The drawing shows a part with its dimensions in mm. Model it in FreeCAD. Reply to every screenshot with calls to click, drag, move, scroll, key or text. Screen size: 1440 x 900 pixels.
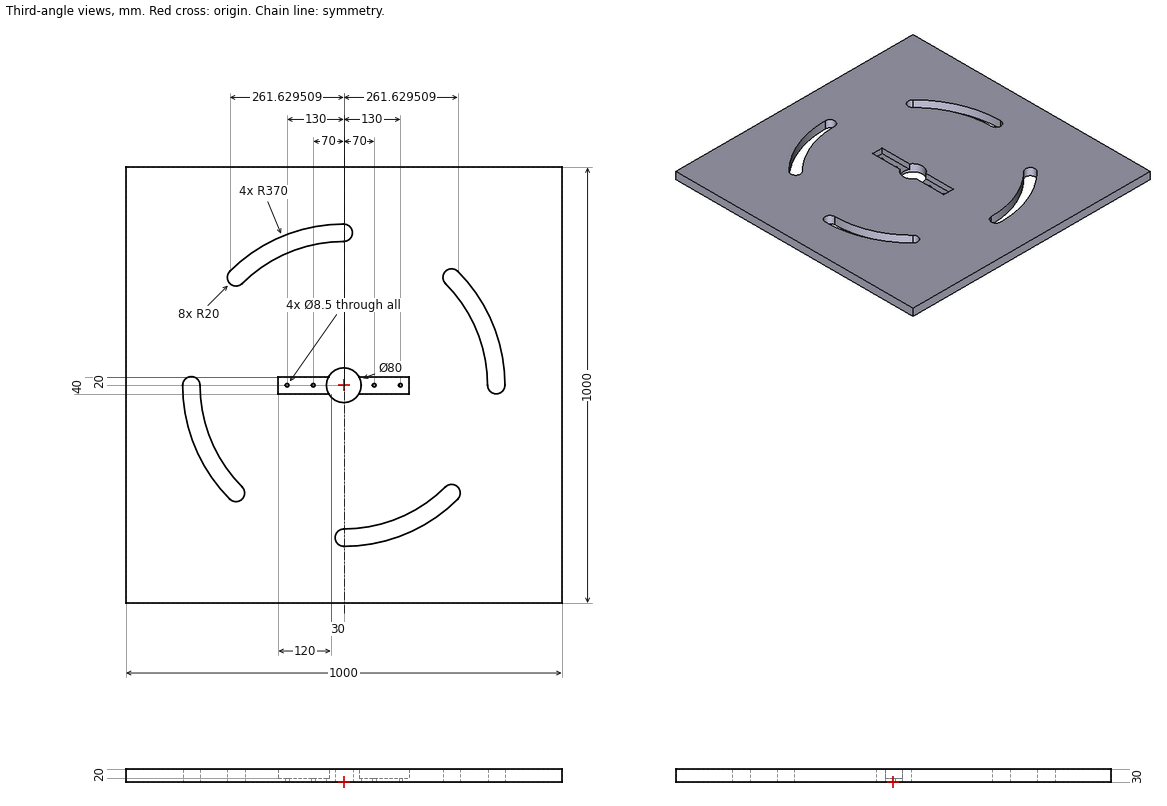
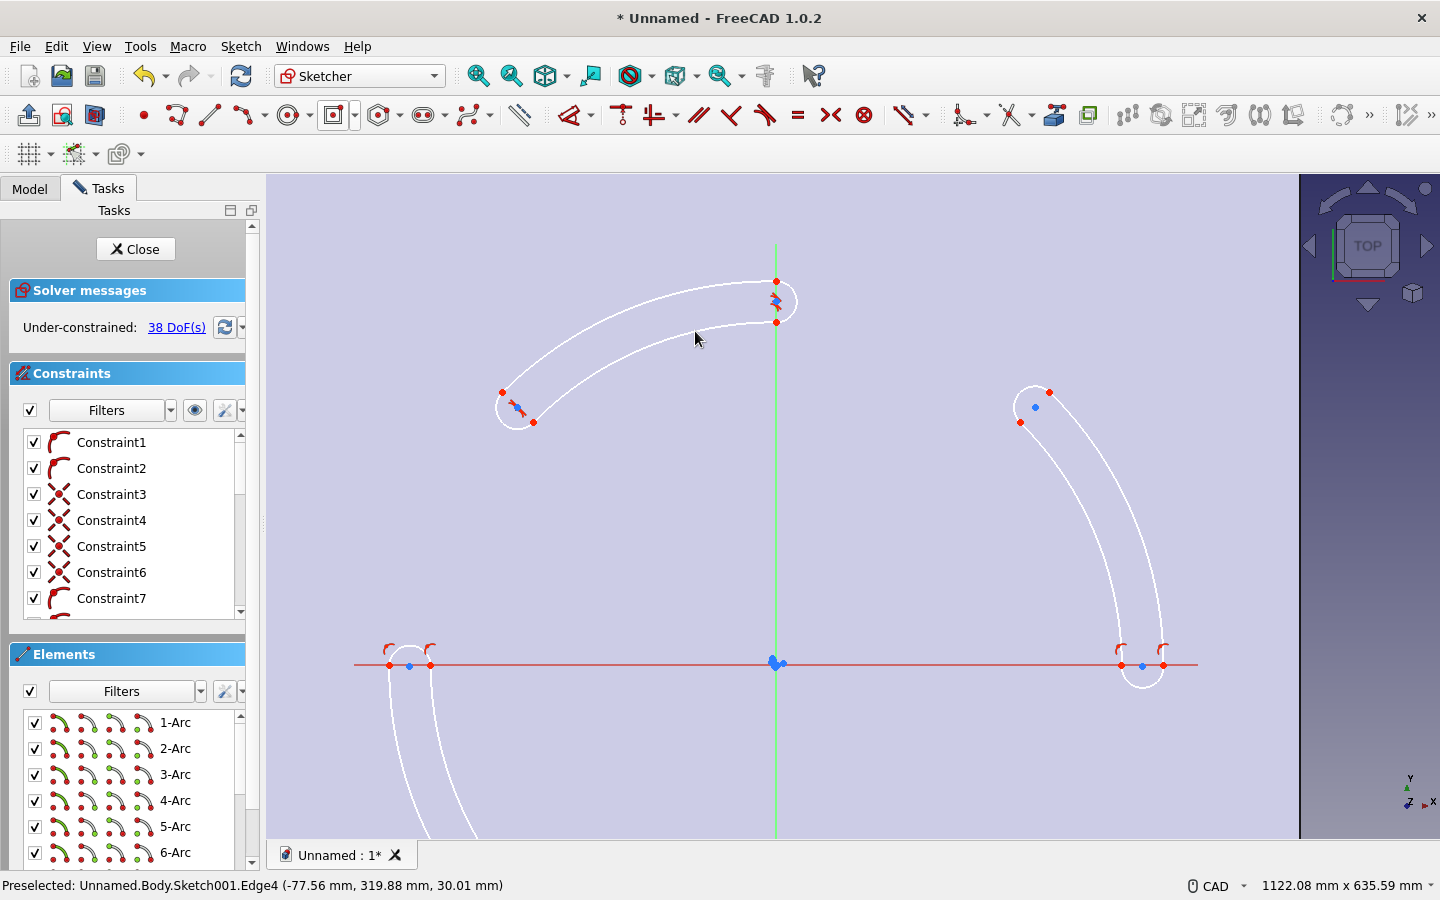
click(1130, 683)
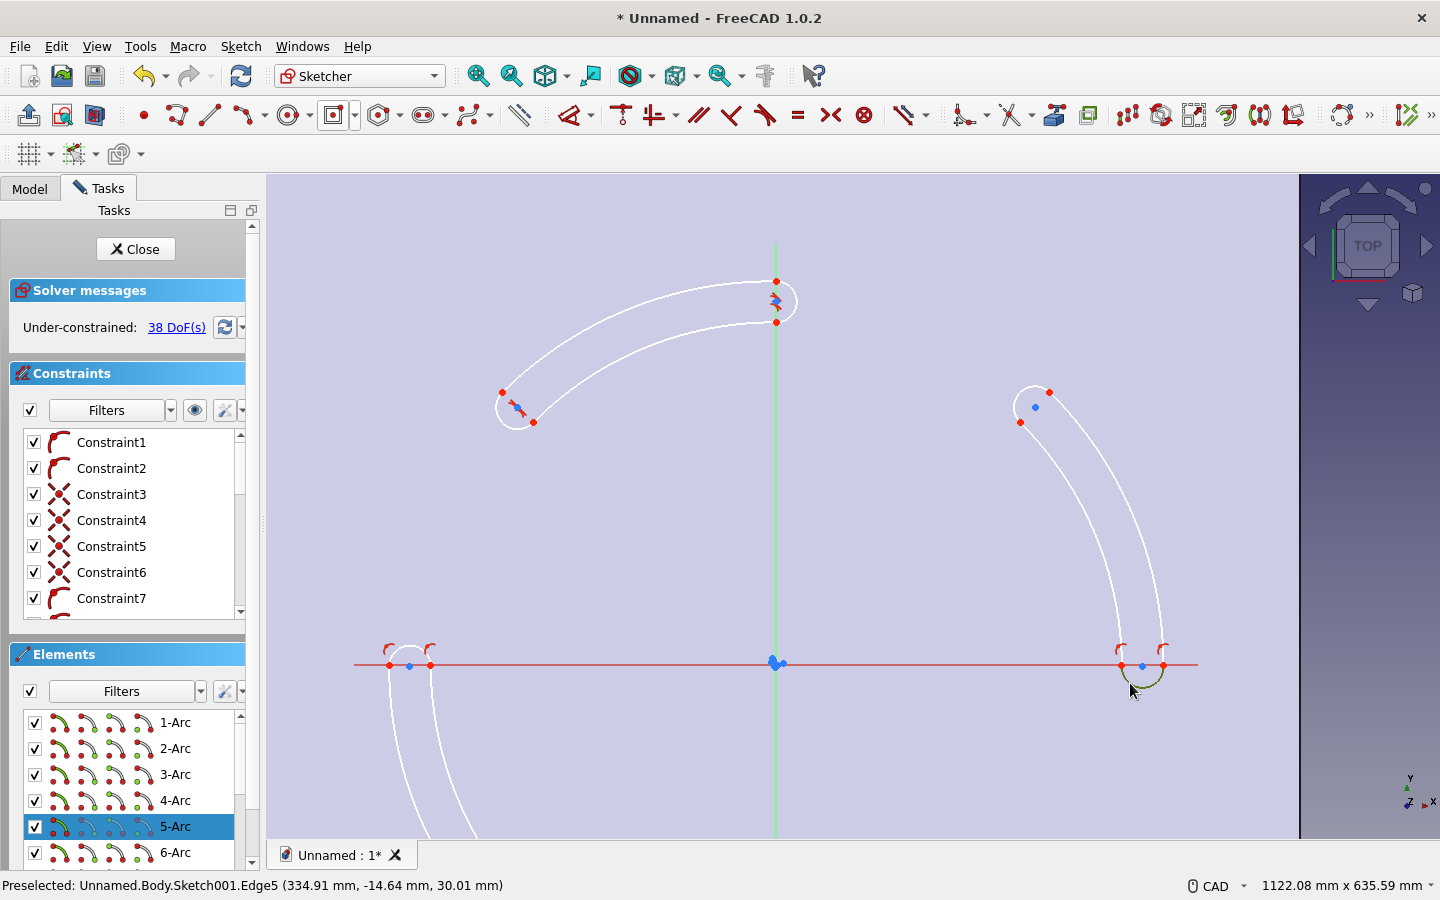
click(1153, 575)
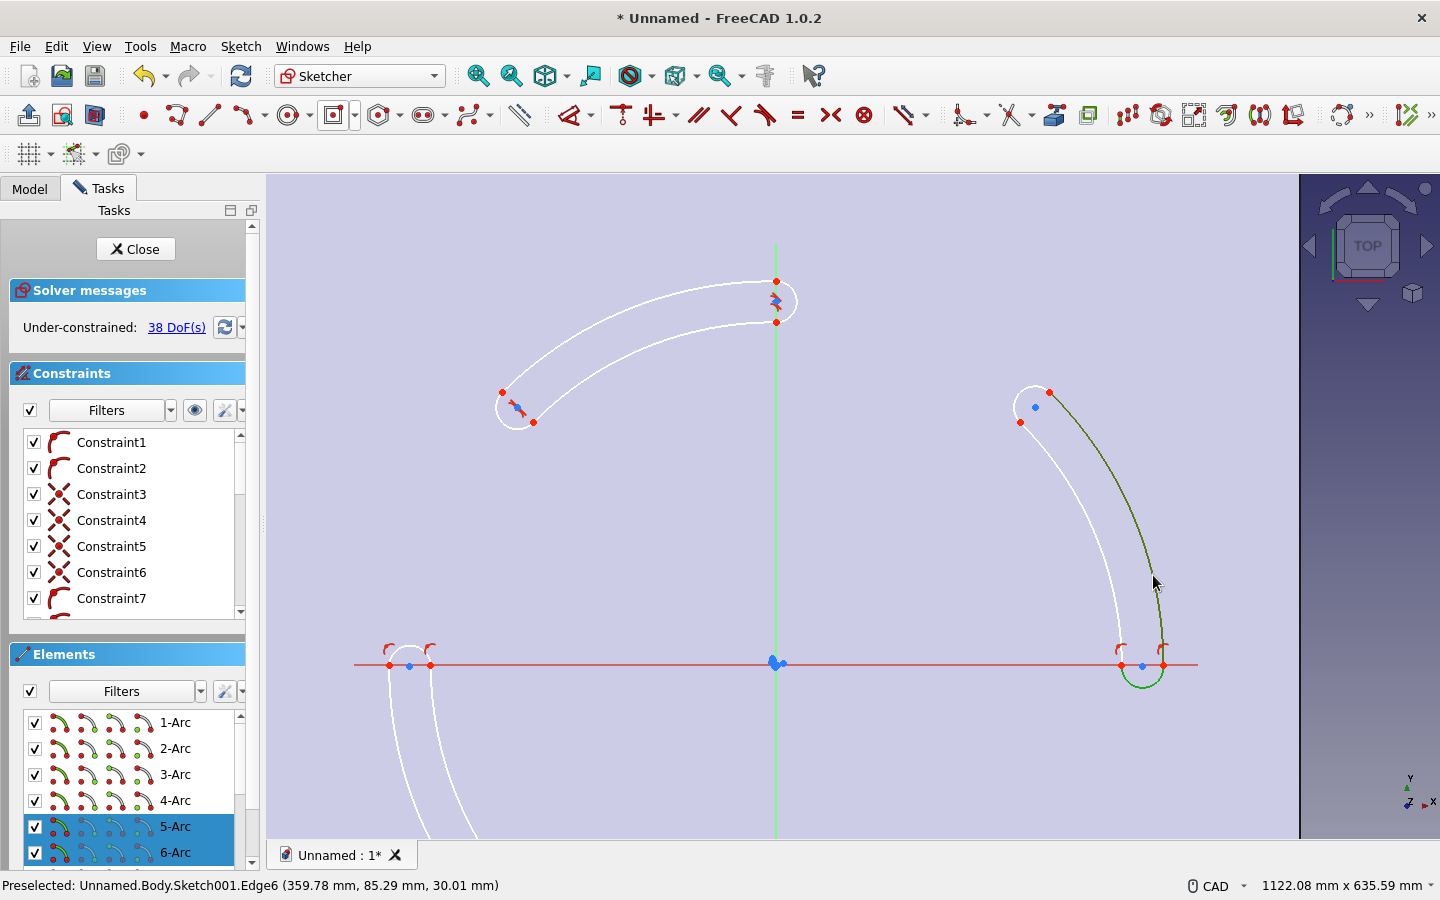
click(765, 116)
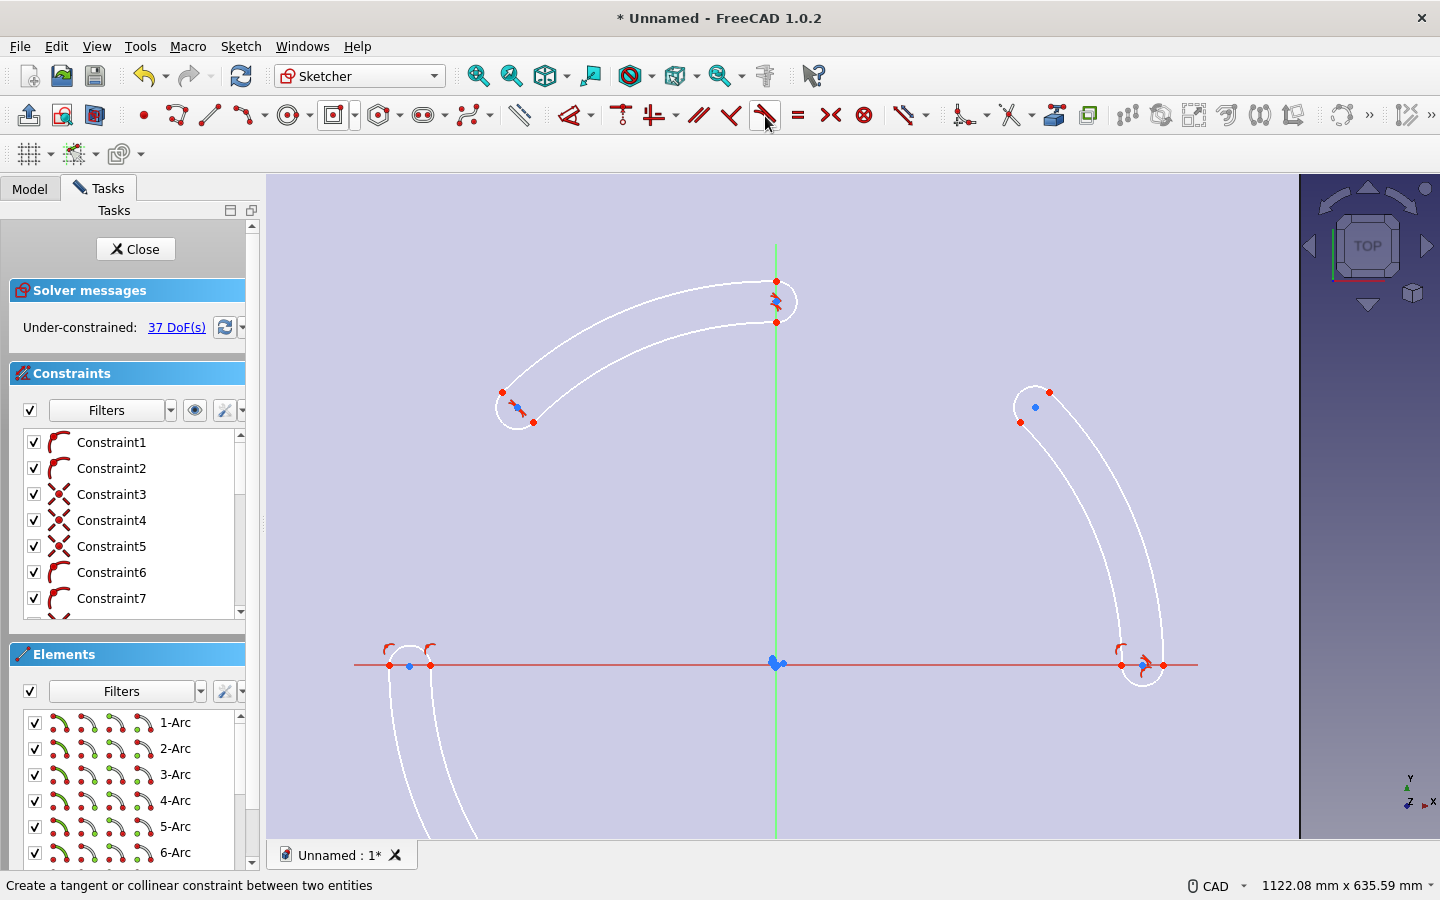
click(1153, 575)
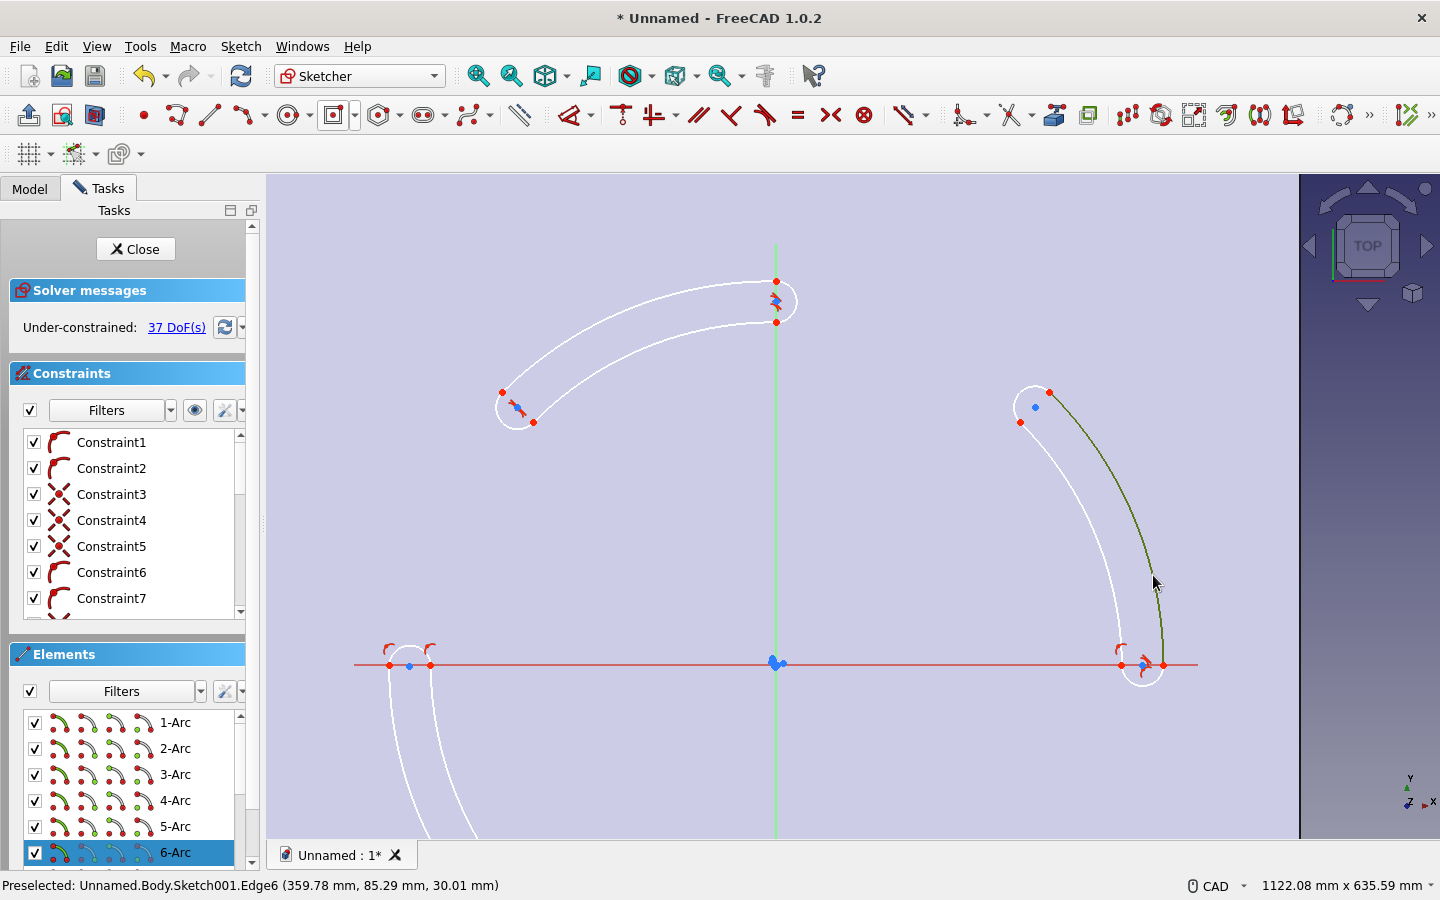
click(1031, 387)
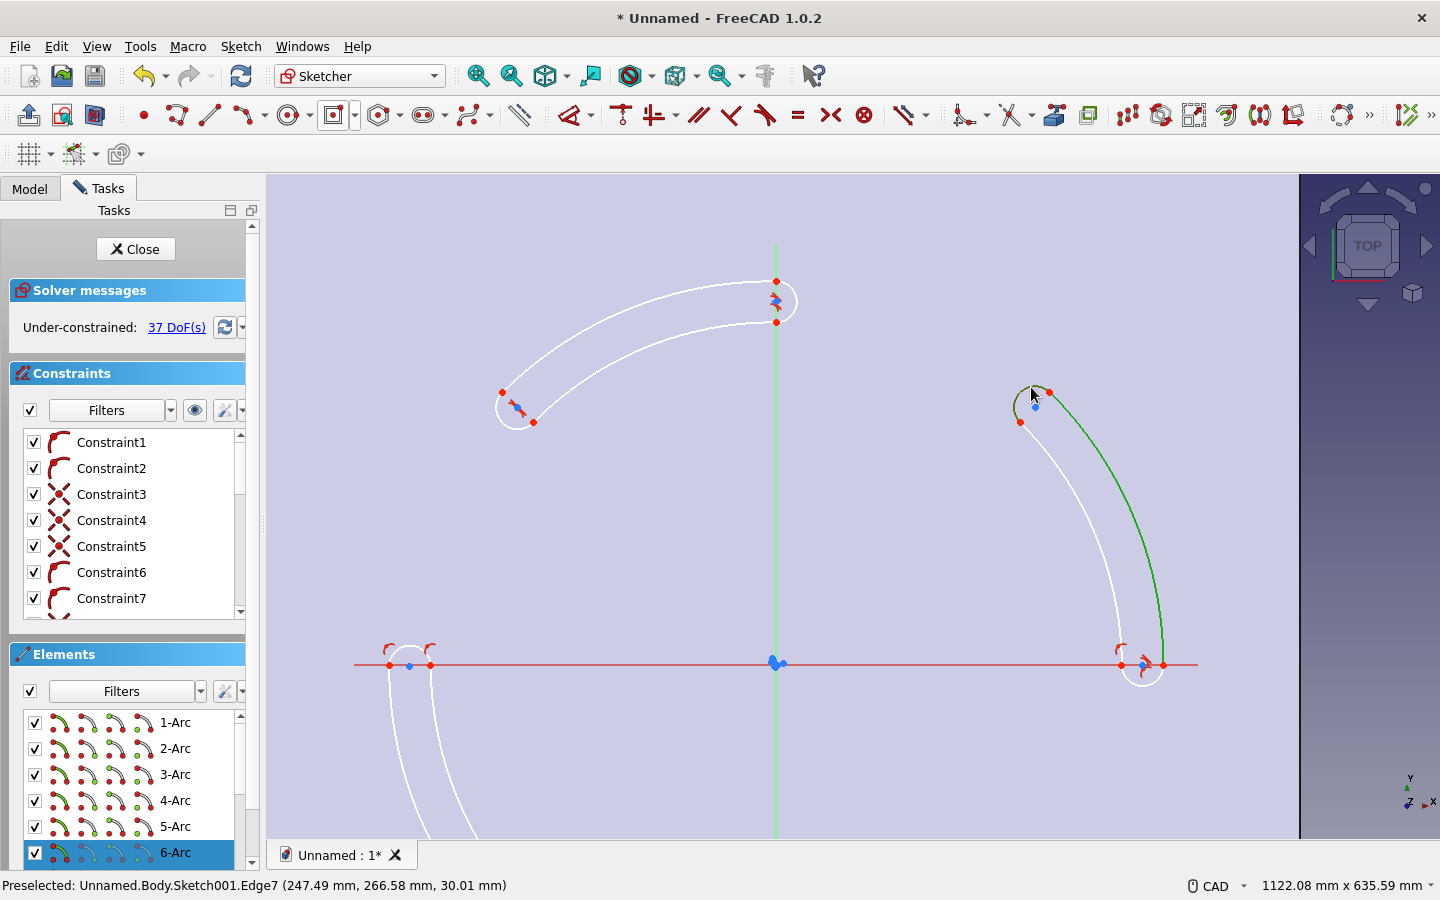
click(765, 116)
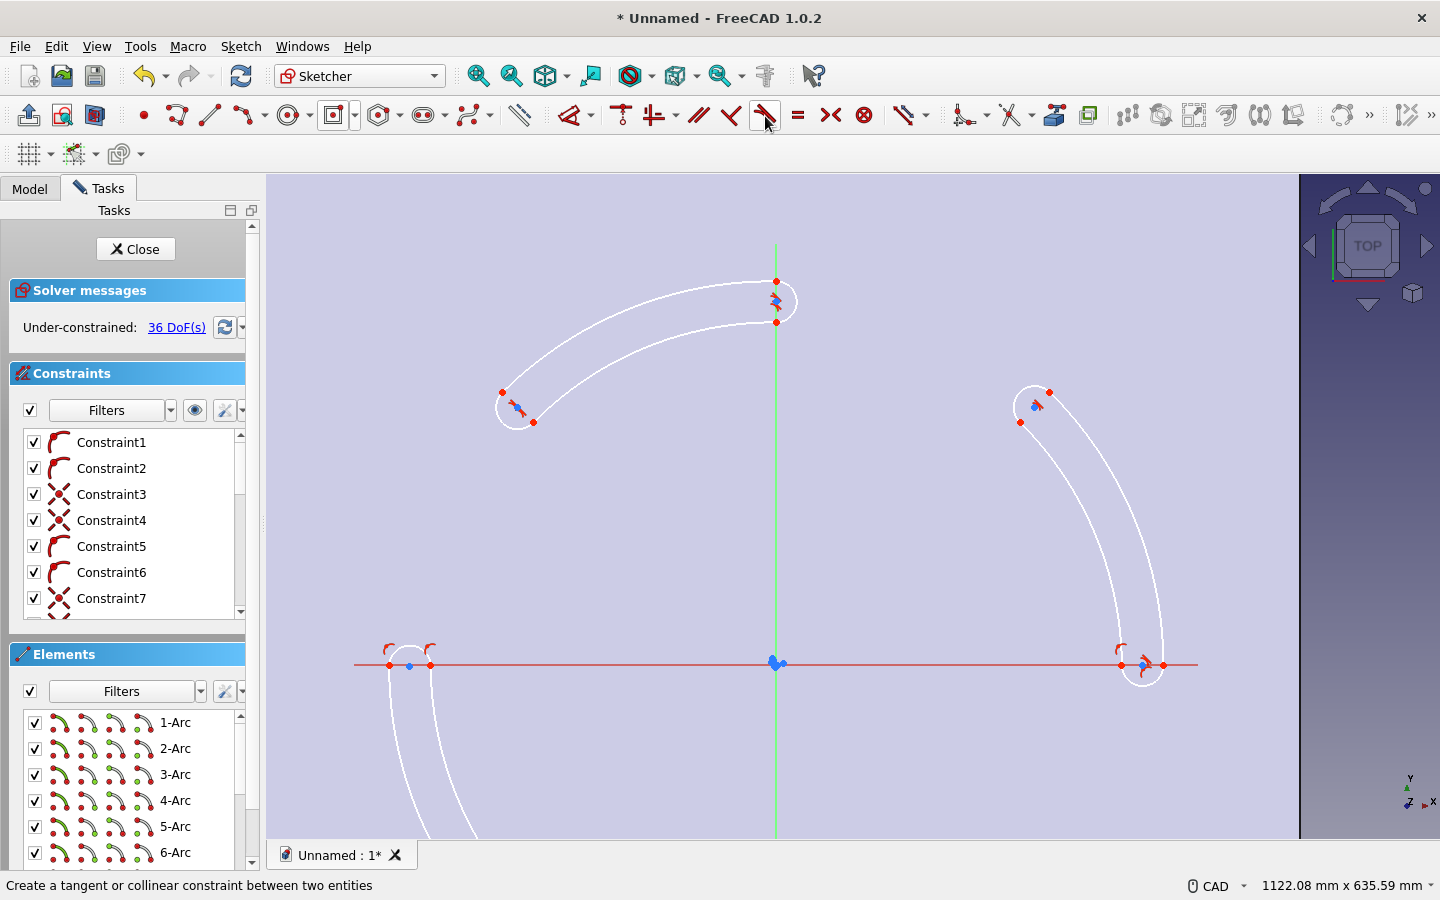
click(1031, 386)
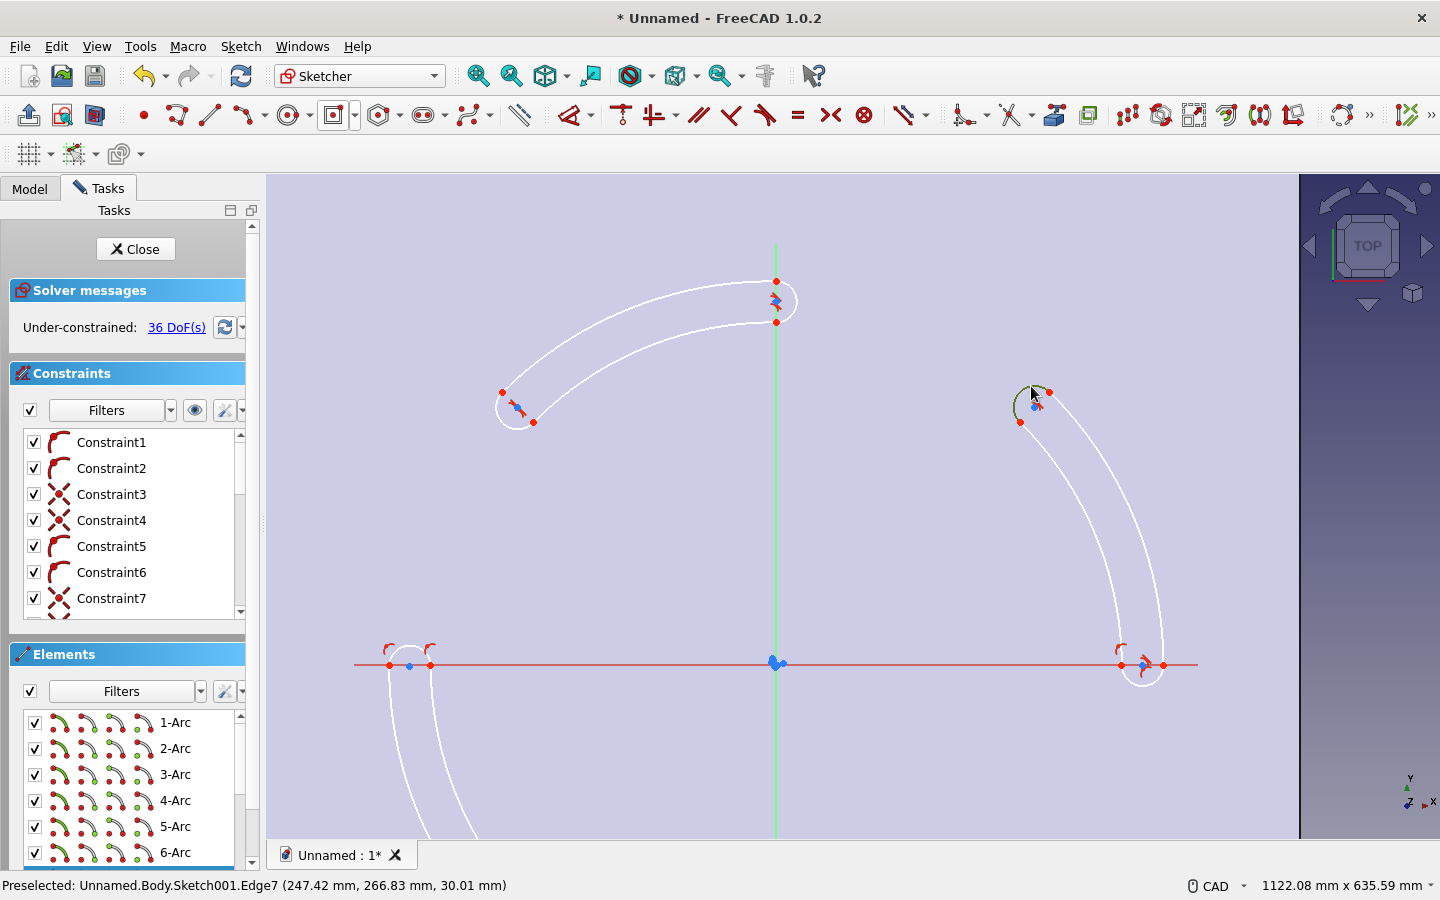
click(1112, 585)